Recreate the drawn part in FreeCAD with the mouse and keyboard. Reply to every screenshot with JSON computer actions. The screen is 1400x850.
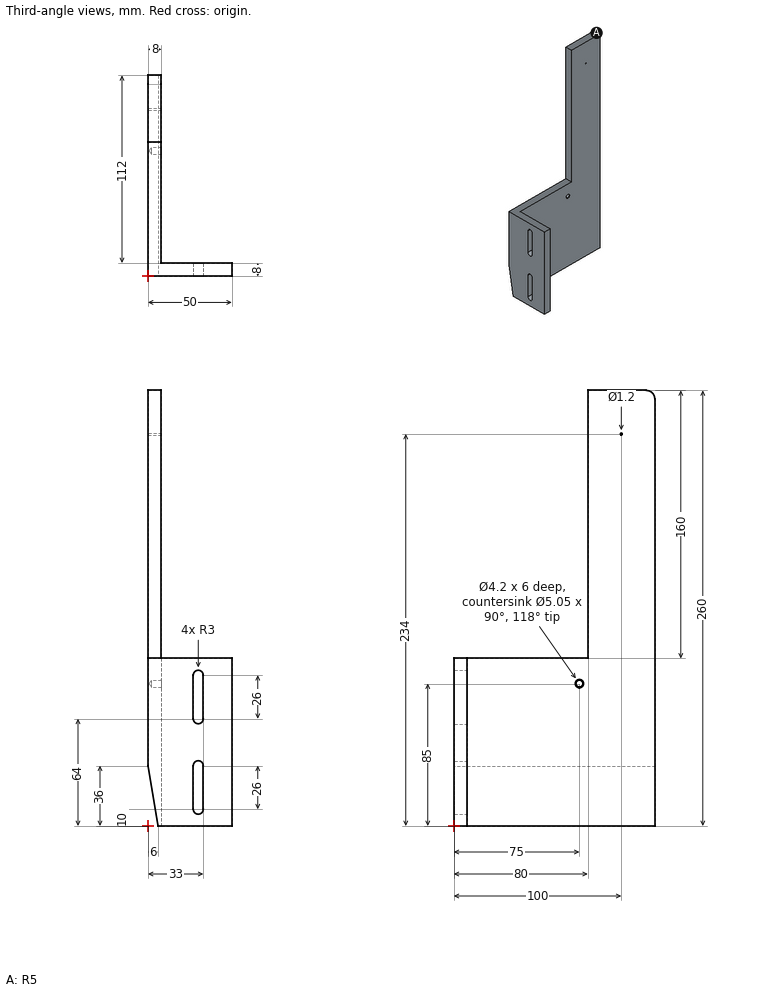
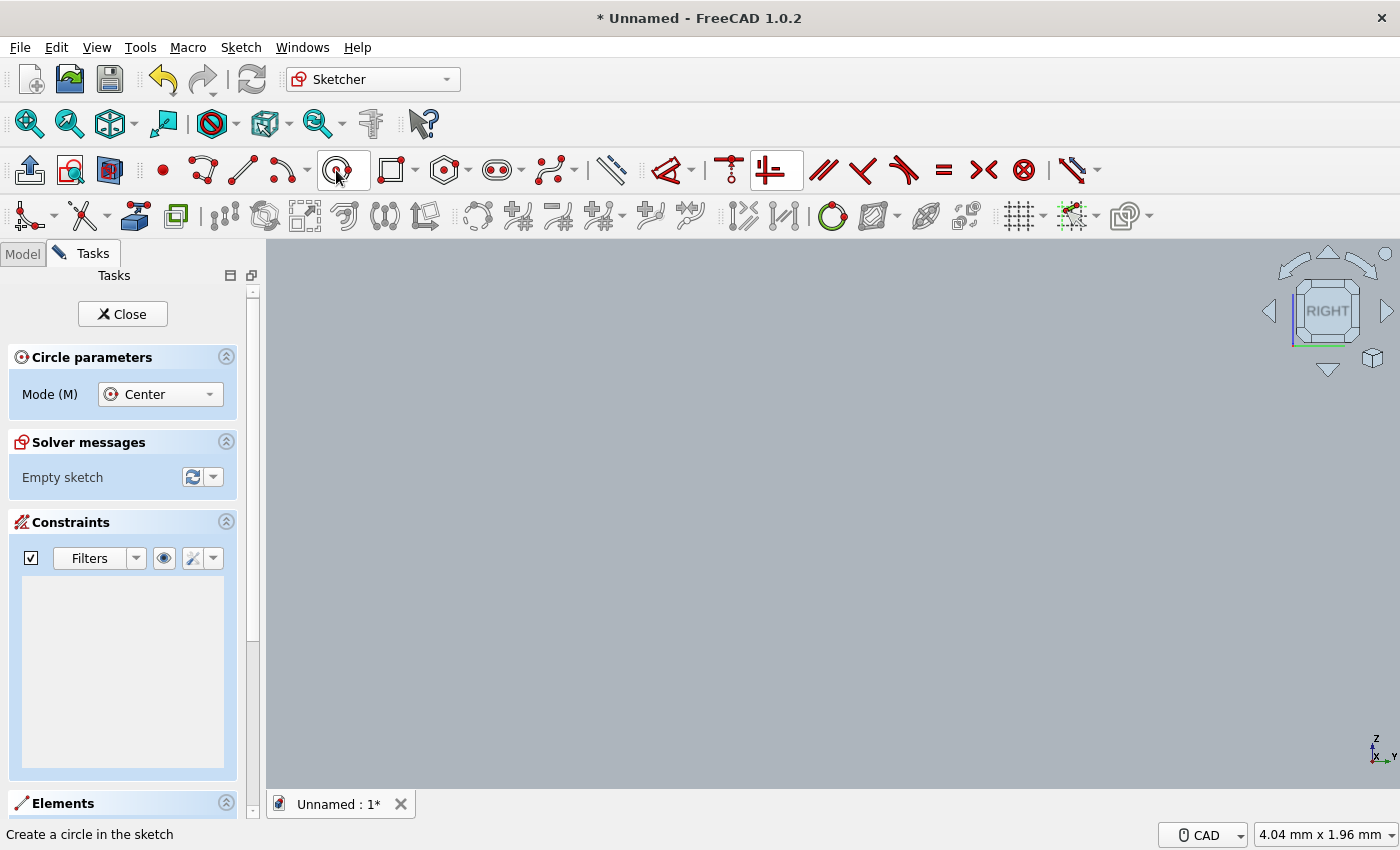
{"action": "left_click", "coordinate": [762, 513]}
{"action": "mouse_move", "coordinate": [881, 394]}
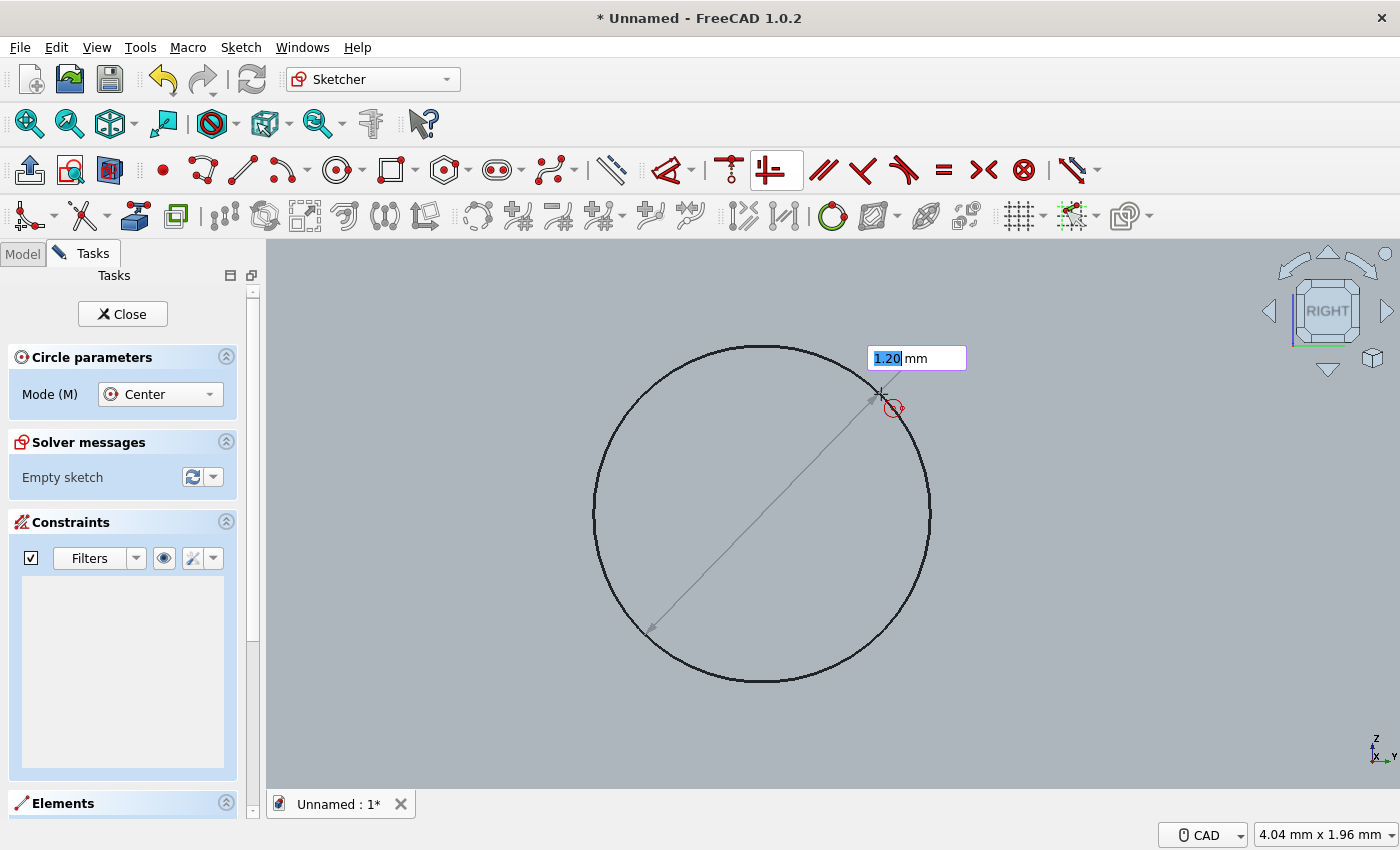
{"action": "type", "text": "1.2"}
{"action": "key", "text": "Return"}
{"action": "key", "text": "Escape"}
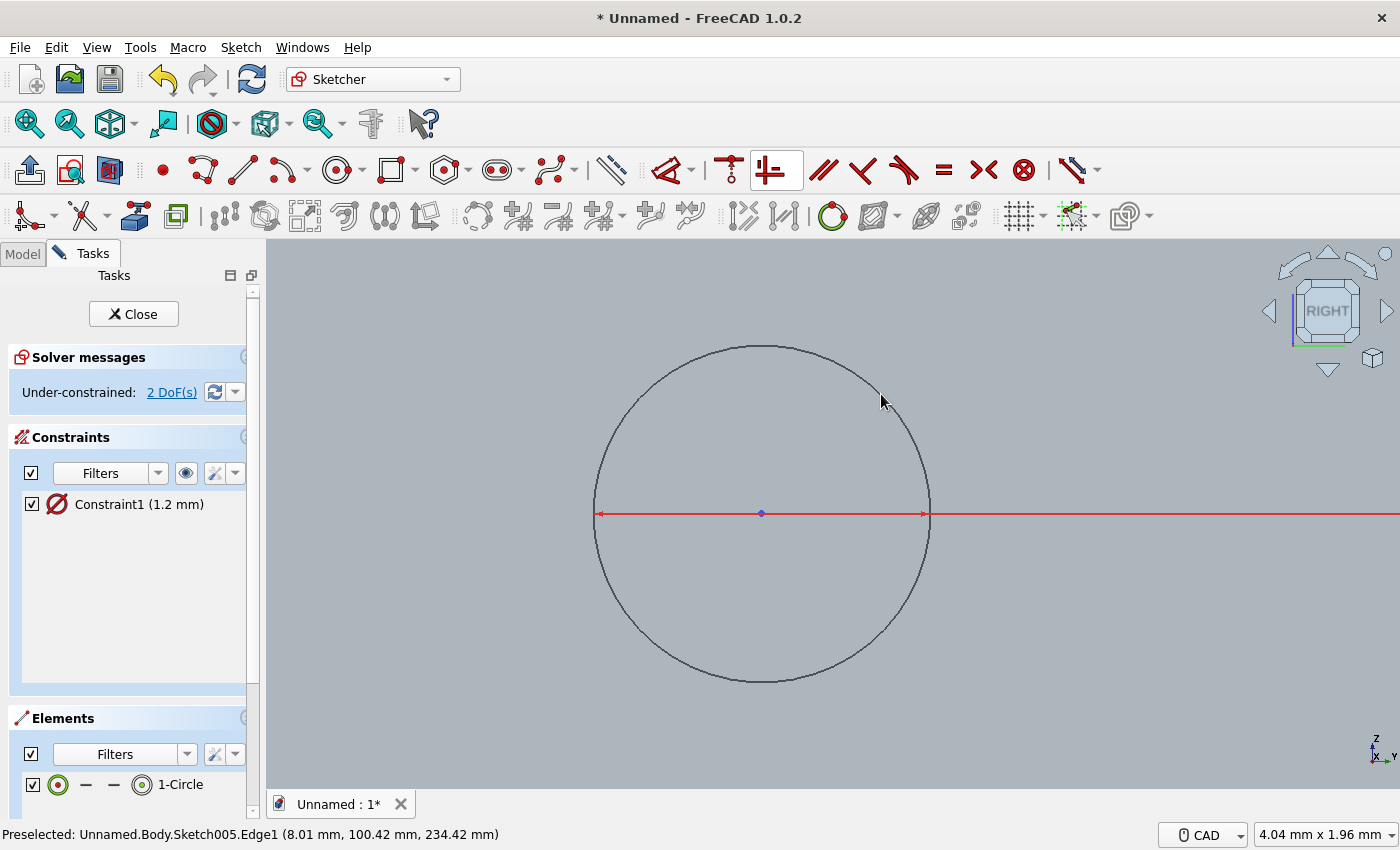
{"action": "left_click", "coordinate": [666, 170]}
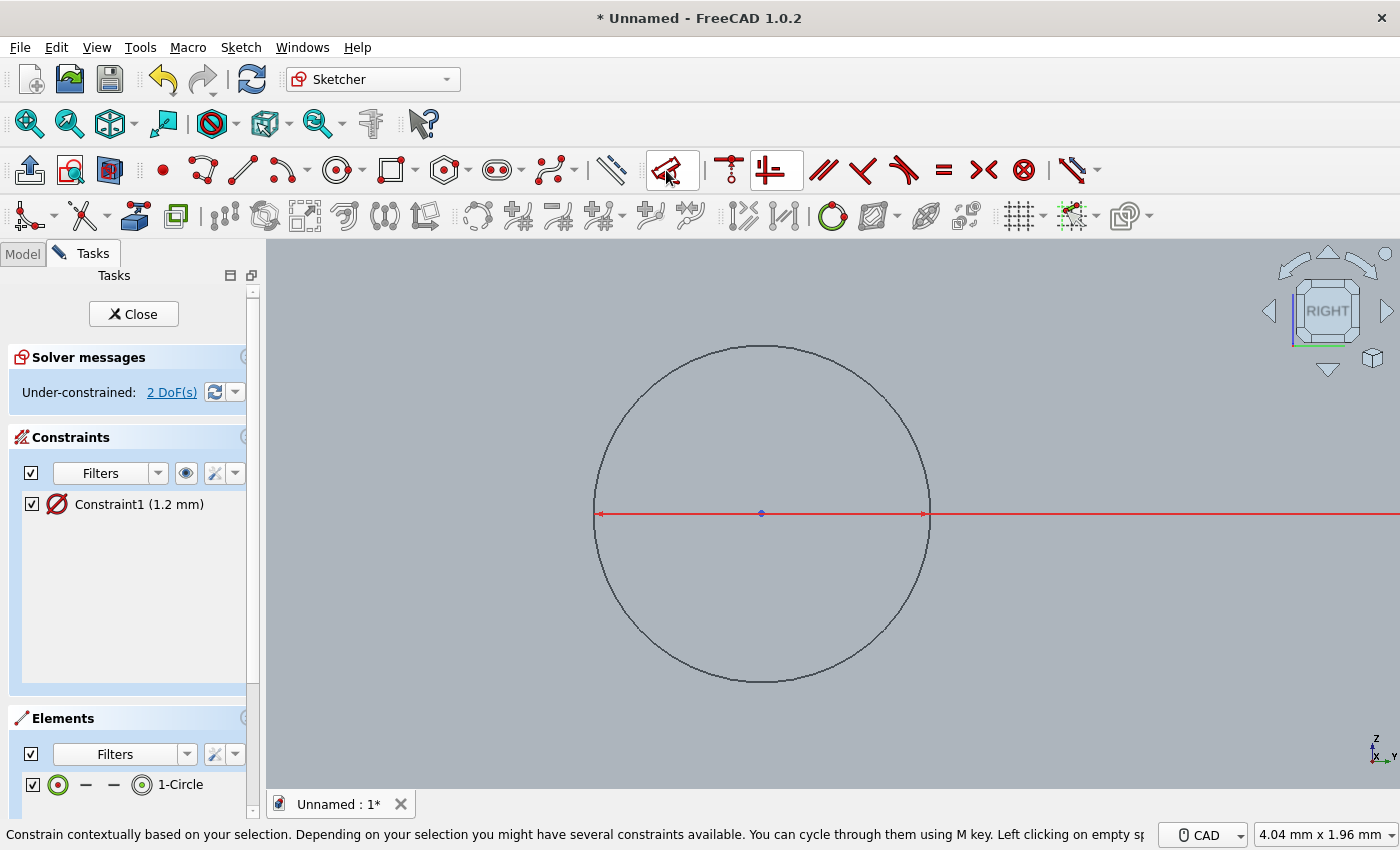
{"action": "left_click", "coordinate": [762, 514]}
{"action": "left_click", "coordinate": [528, 480]}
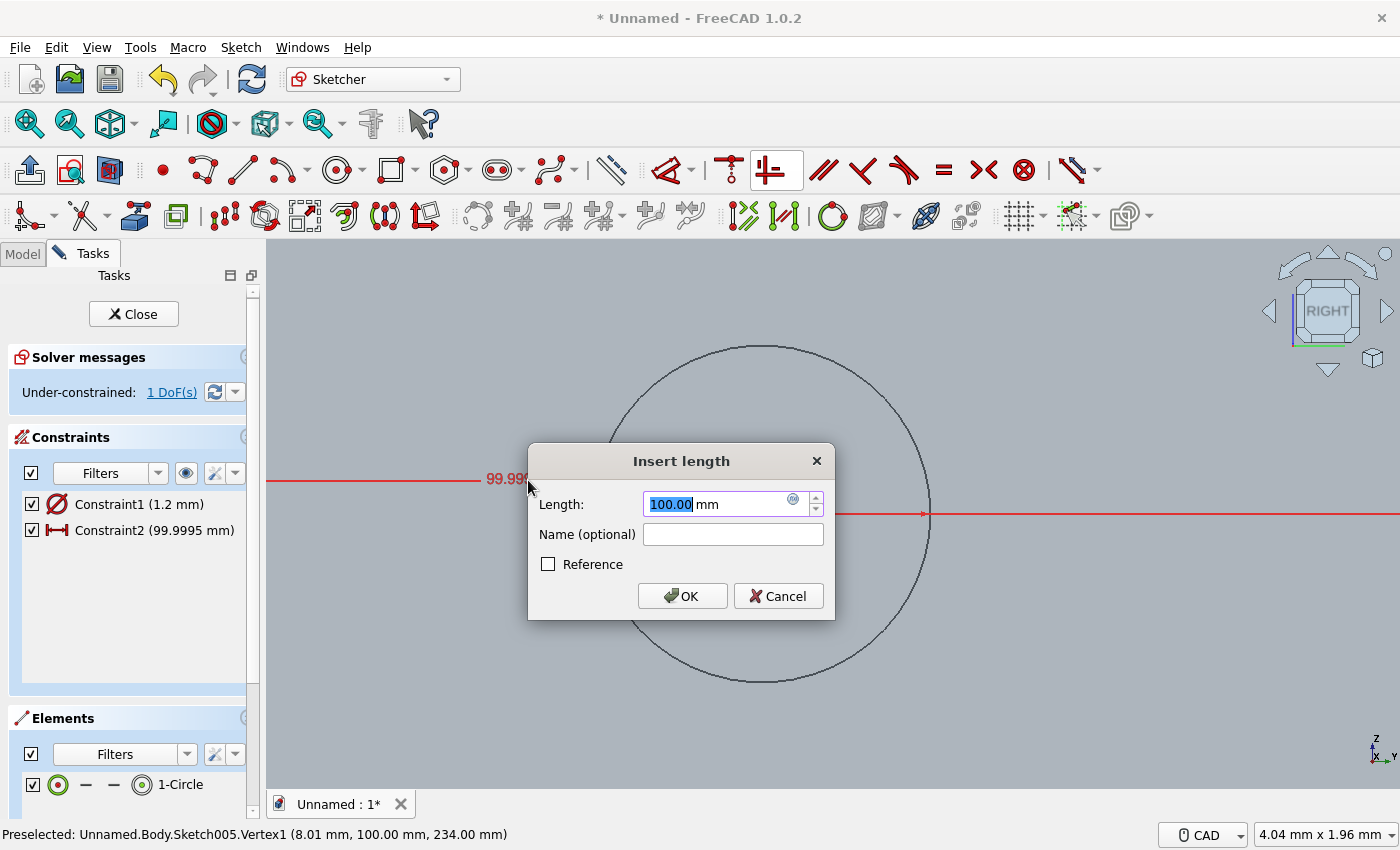
{"action": "type", "text": "100"}
{"action": "key", "text": "Return"}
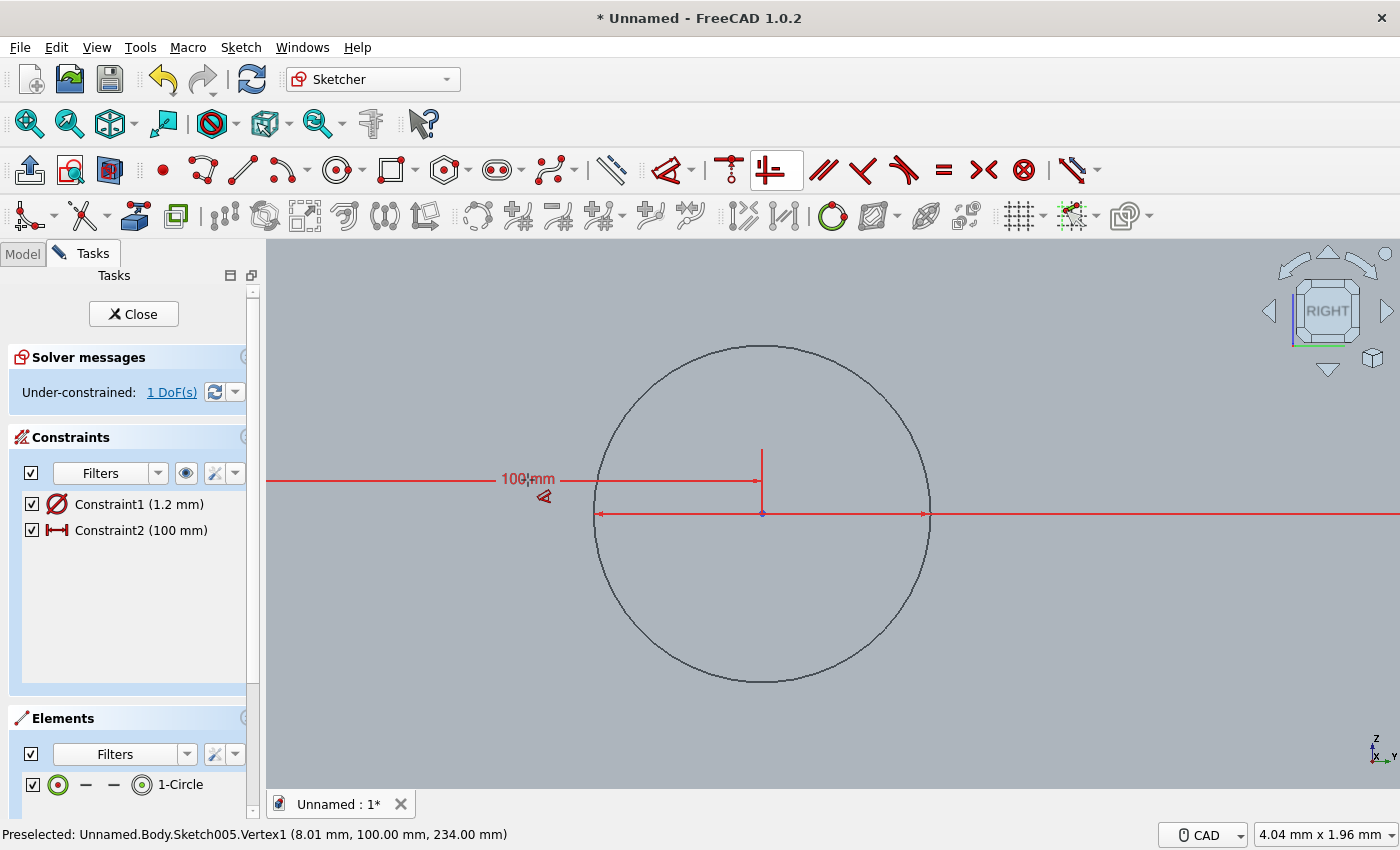
{"action": "left_click", "coordinate": [762, 514]}
{"action": "left_click", "coordinate": [796, 637]}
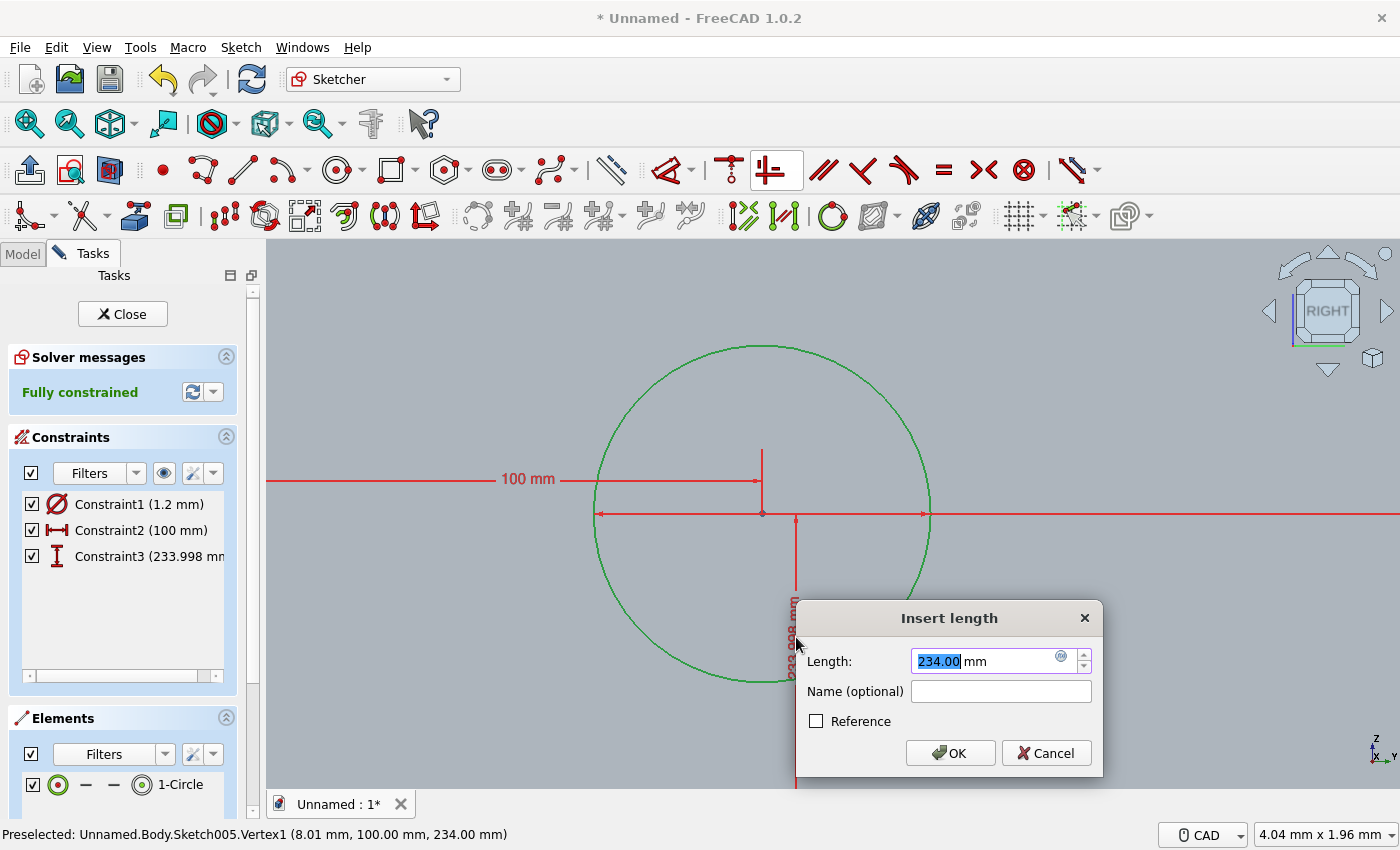
{"action": "type", "text": "234"}
{"action": "key", "text": "Return"}
{"action": "key", "text": "Escape"}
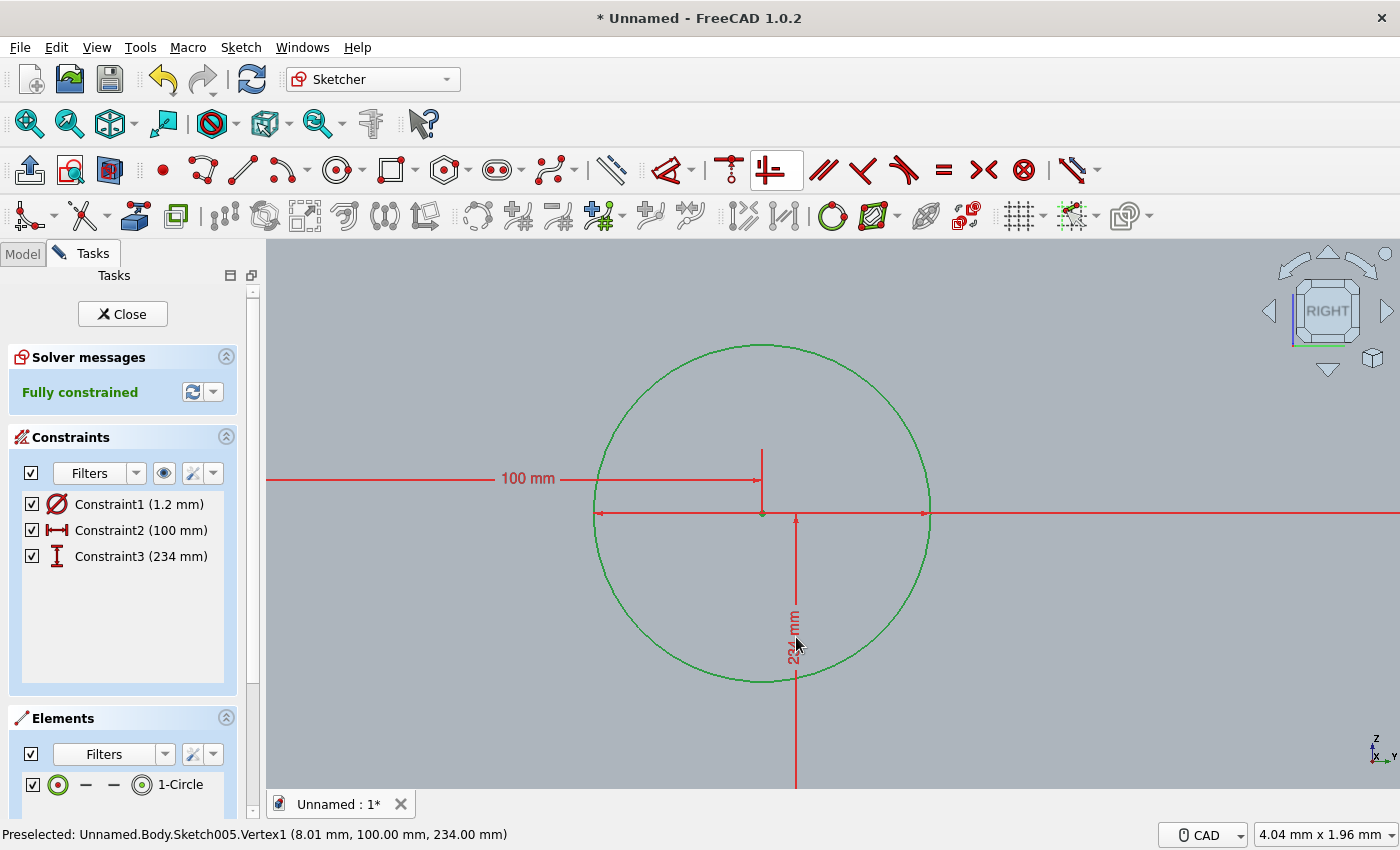
{"action": "left_click", "coordinate": [123, 314]}